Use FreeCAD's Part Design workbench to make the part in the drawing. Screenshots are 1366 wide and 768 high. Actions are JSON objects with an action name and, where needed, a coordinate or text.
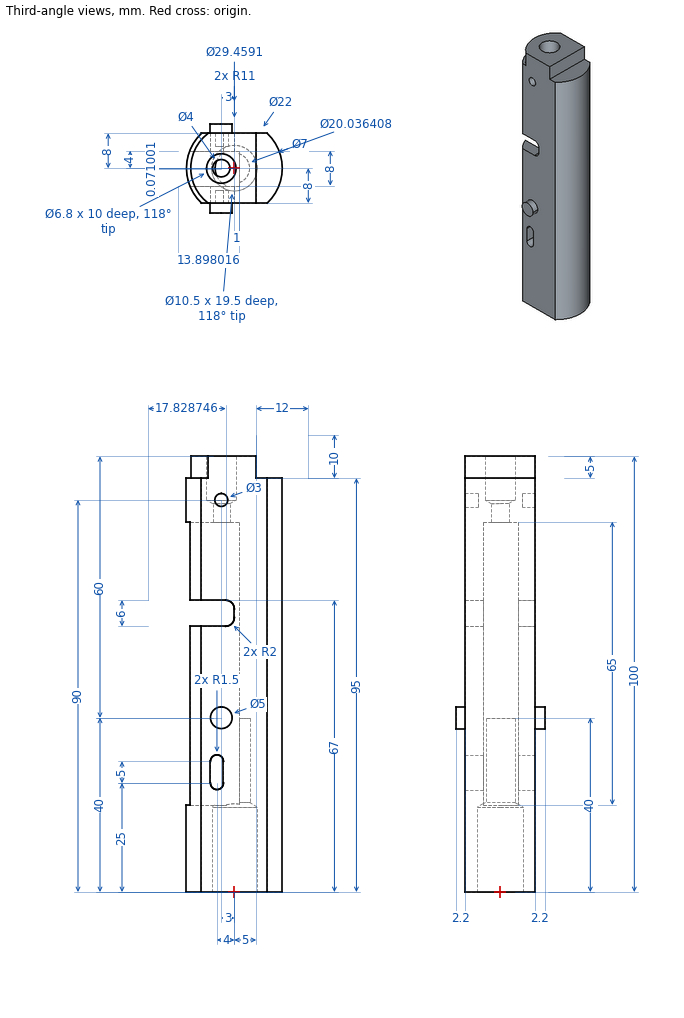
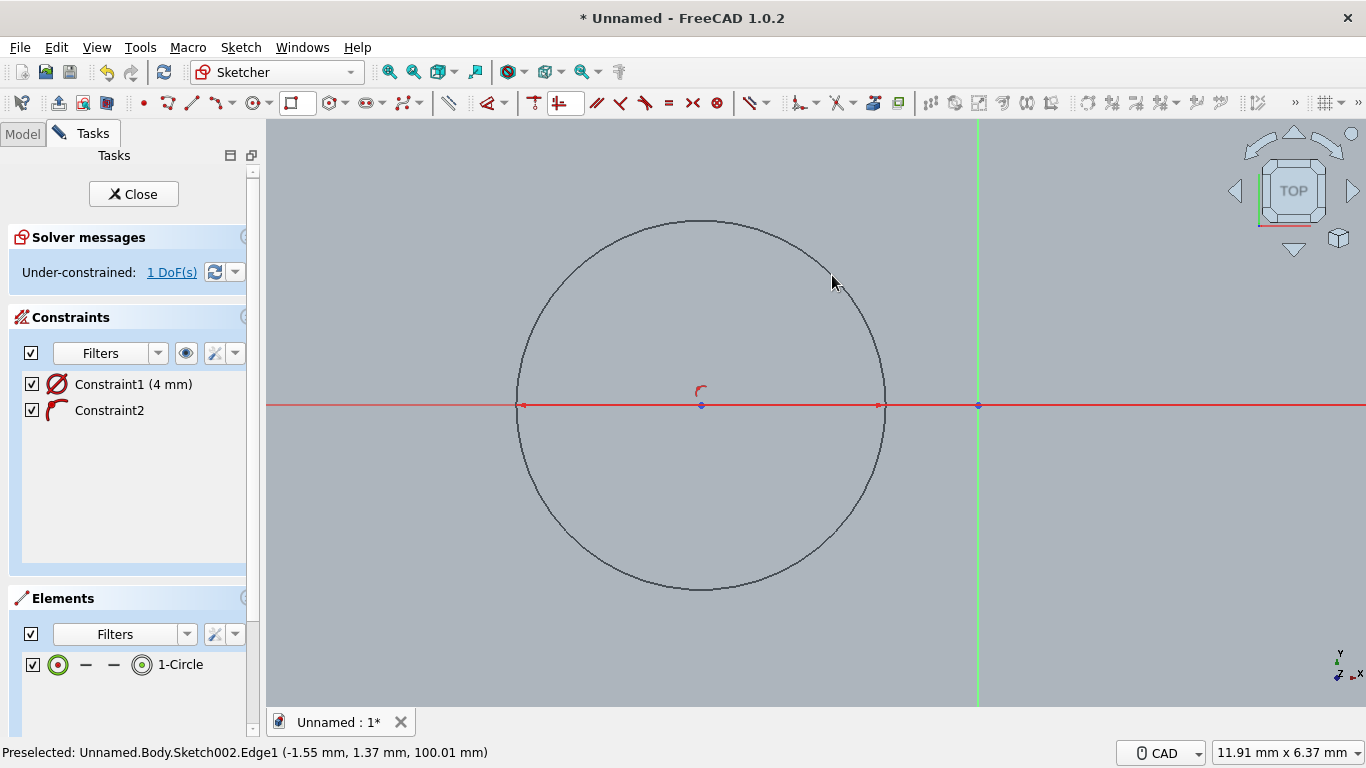
{"action": "key", "text": "d"}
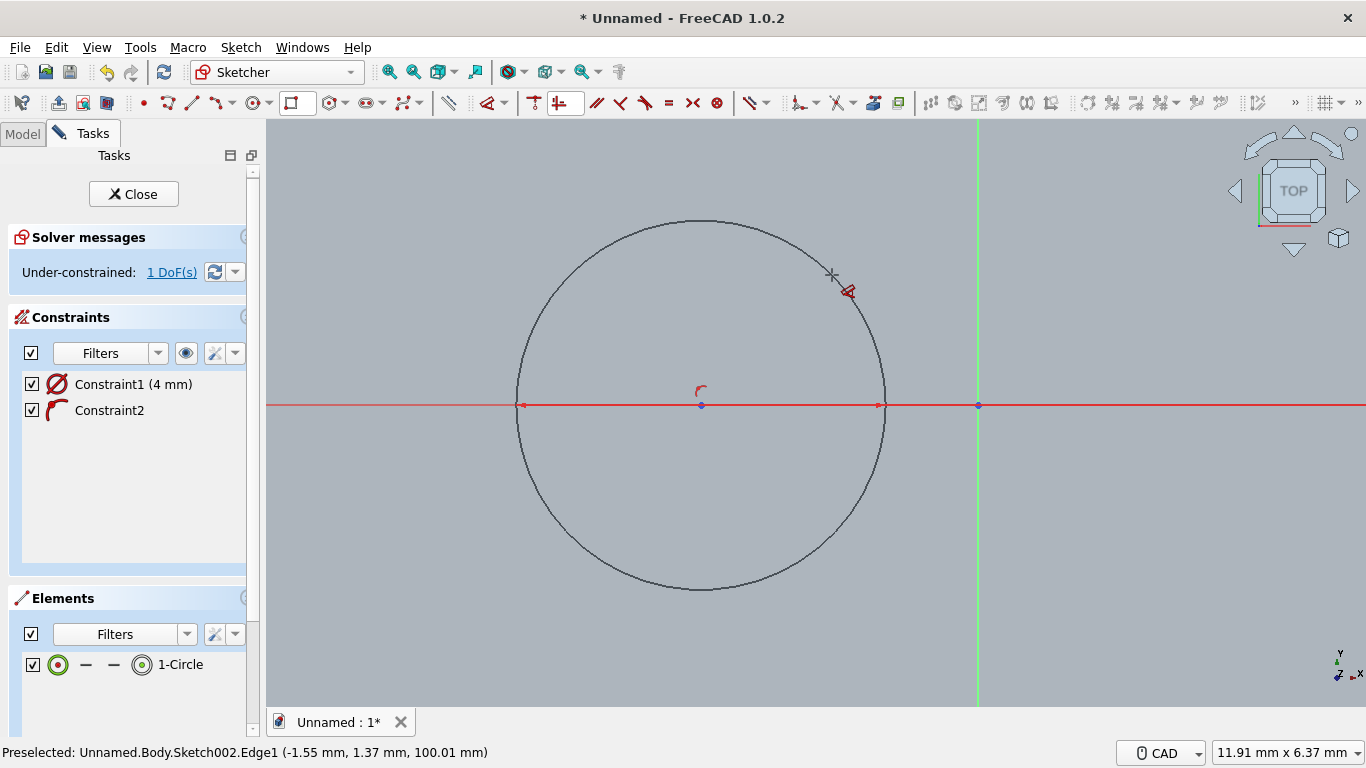
{"action": "left_click", "coordinate": [701, 405]}
{"action": "left_click", "coordinate": [840, 439]}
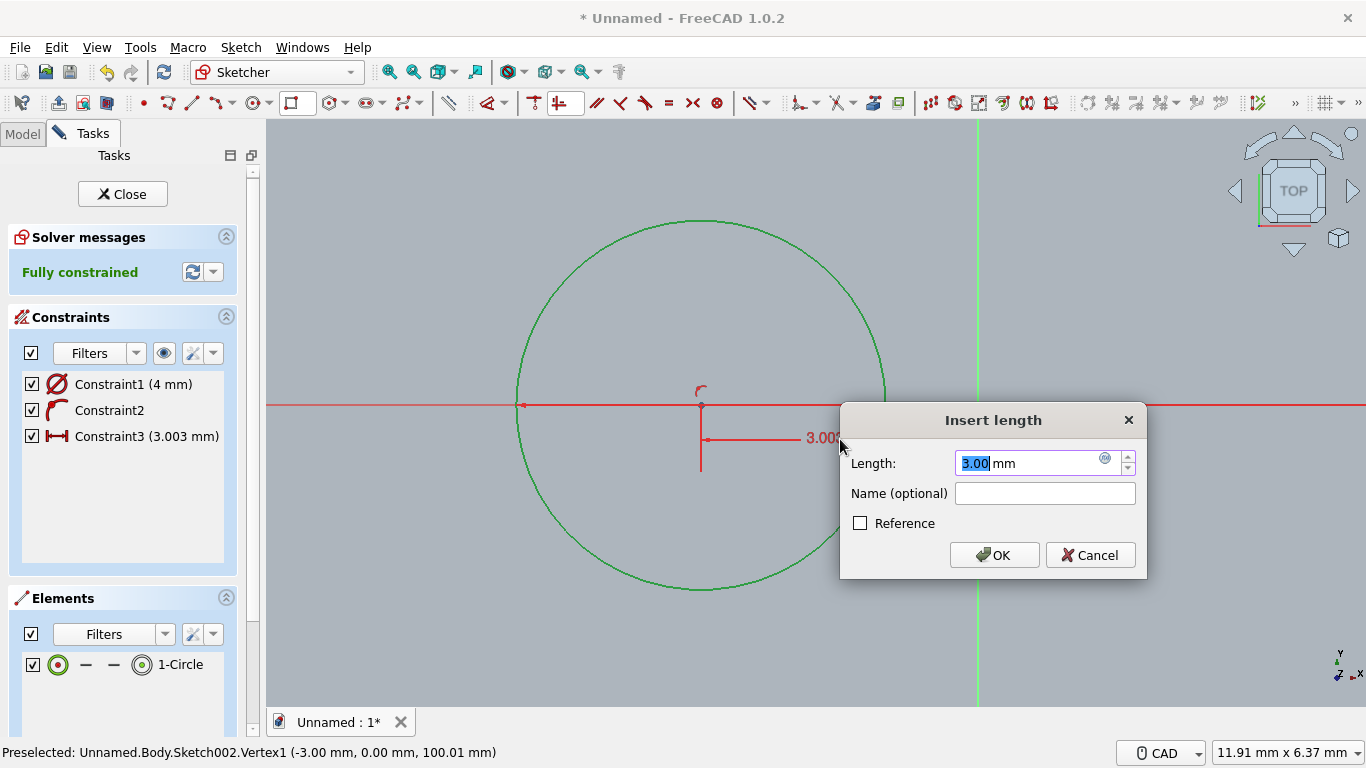
{"action": "type", "text": "3"}
{"action": "key", "text": "Return"}
{"action": "key", "text": "Escape"}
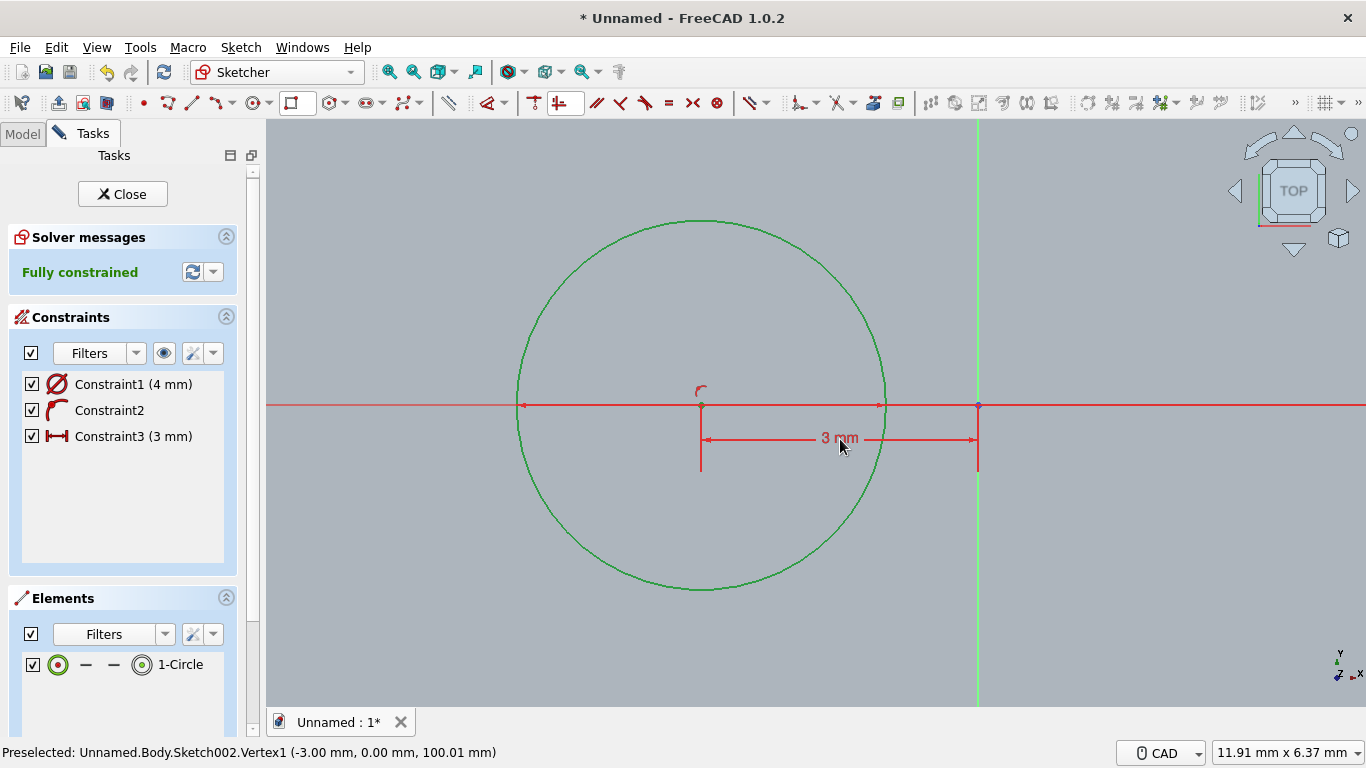
{"action": "left_click", "coordinate": [123, 194]}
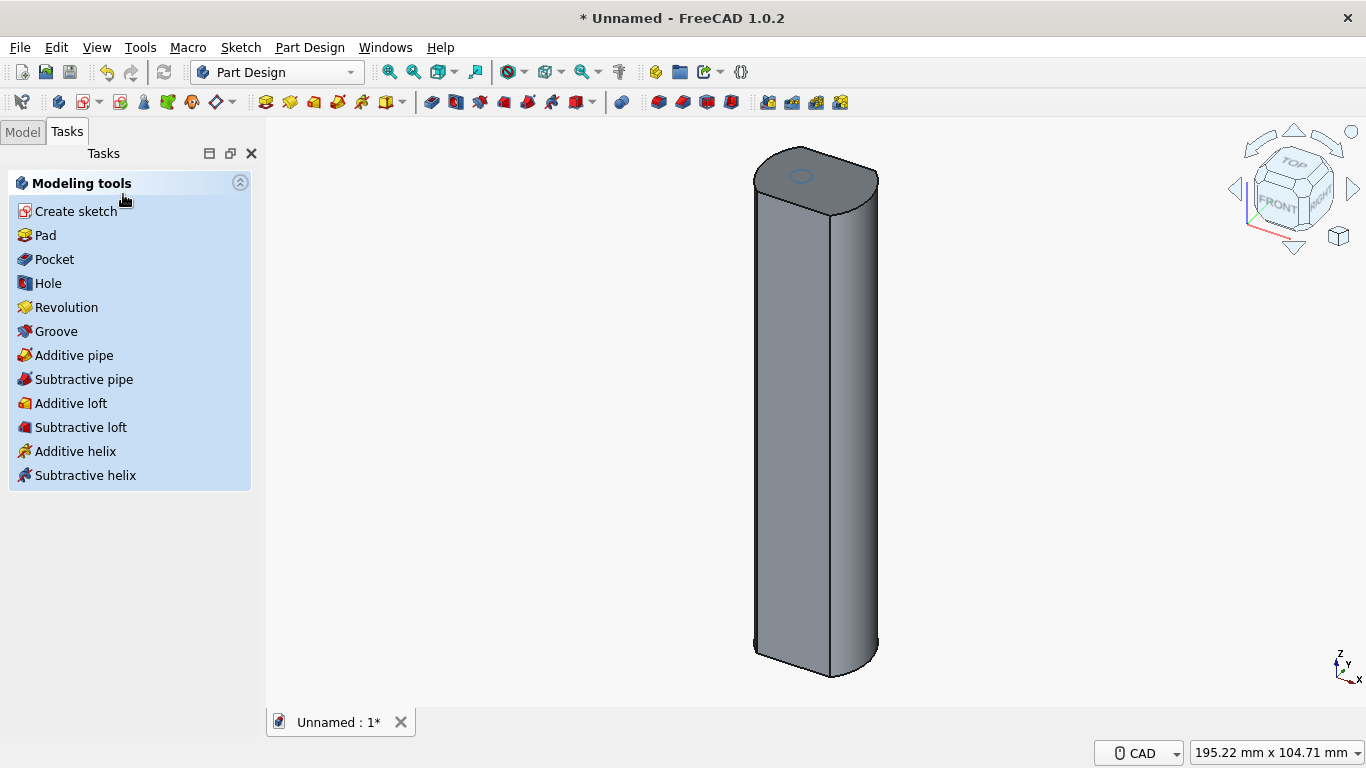
{"action": "left_click", "coordinate": [432, 102]}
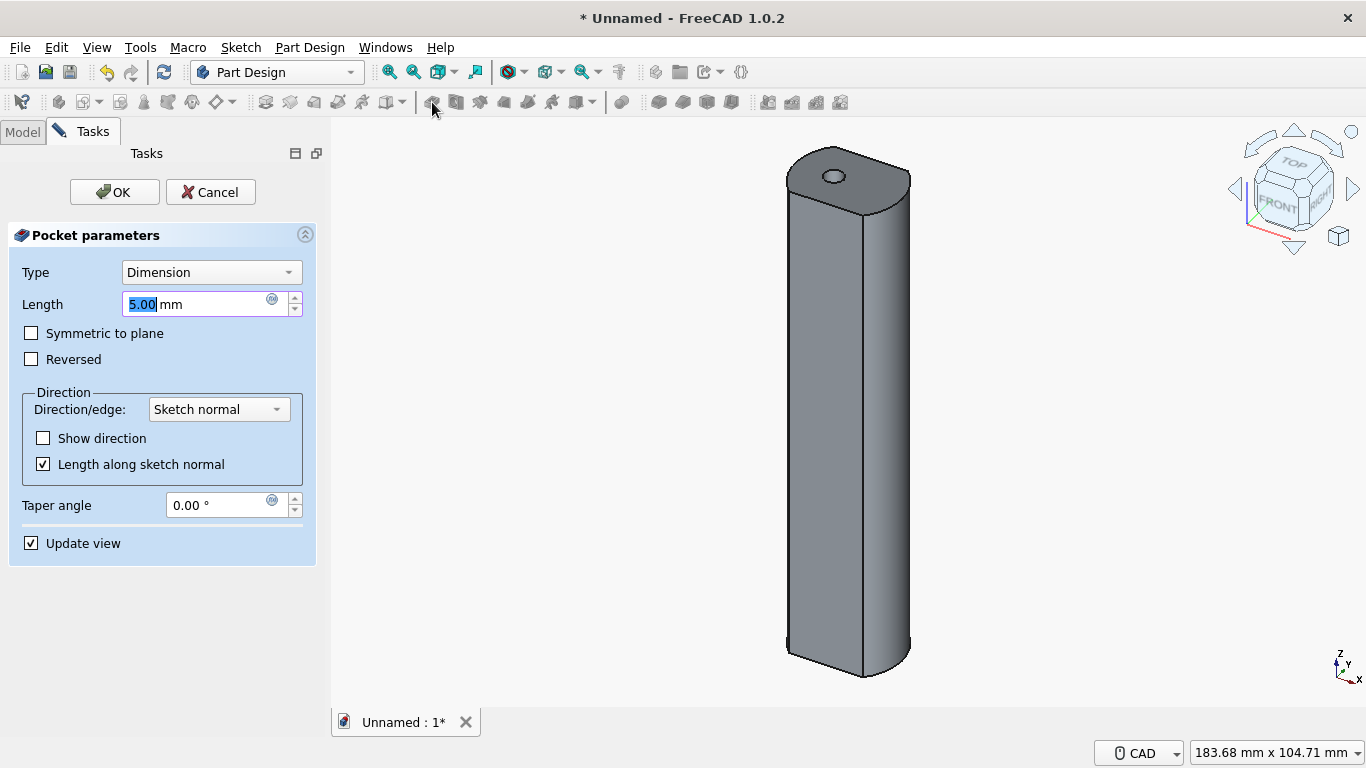
{"action": "type", "text": "60"}
{"action": "key", "text": "Tab"}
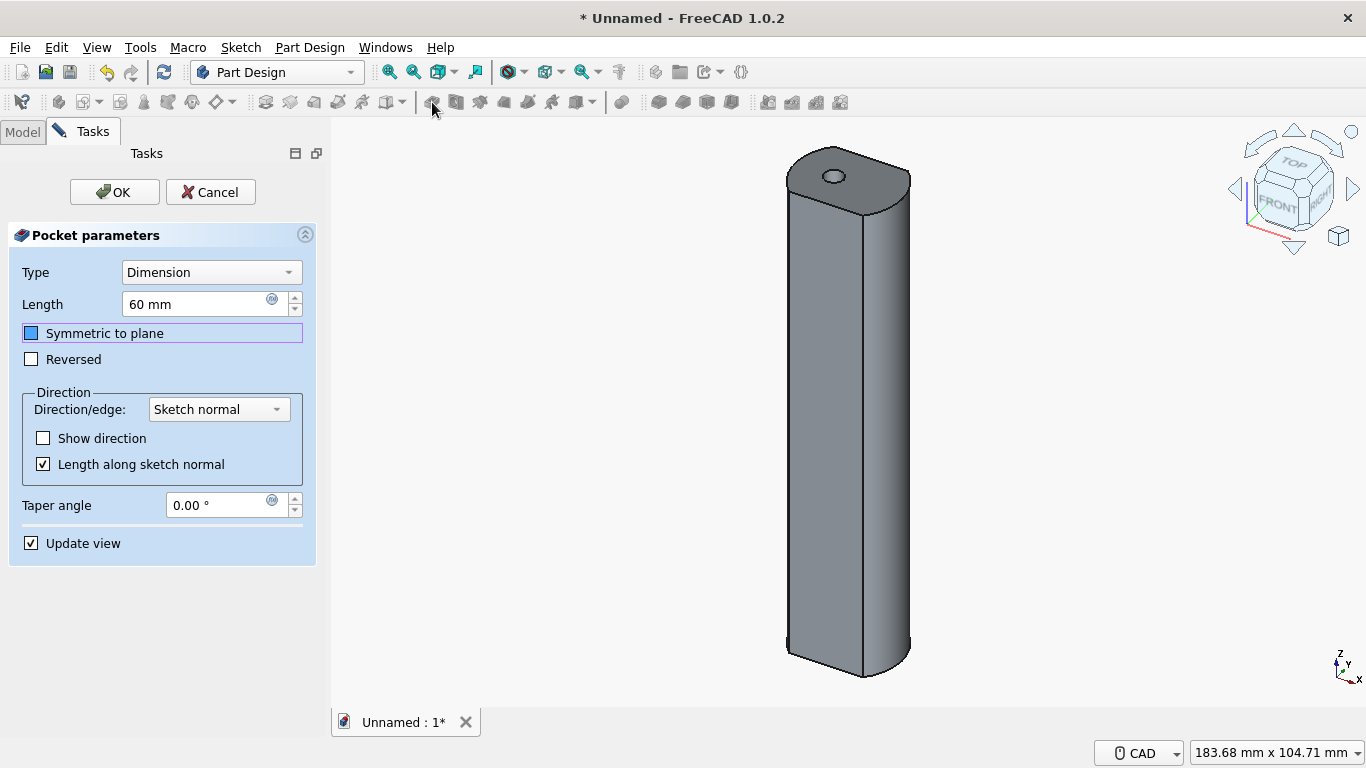
{"action": "left_click", "coordinate": [115, 192]}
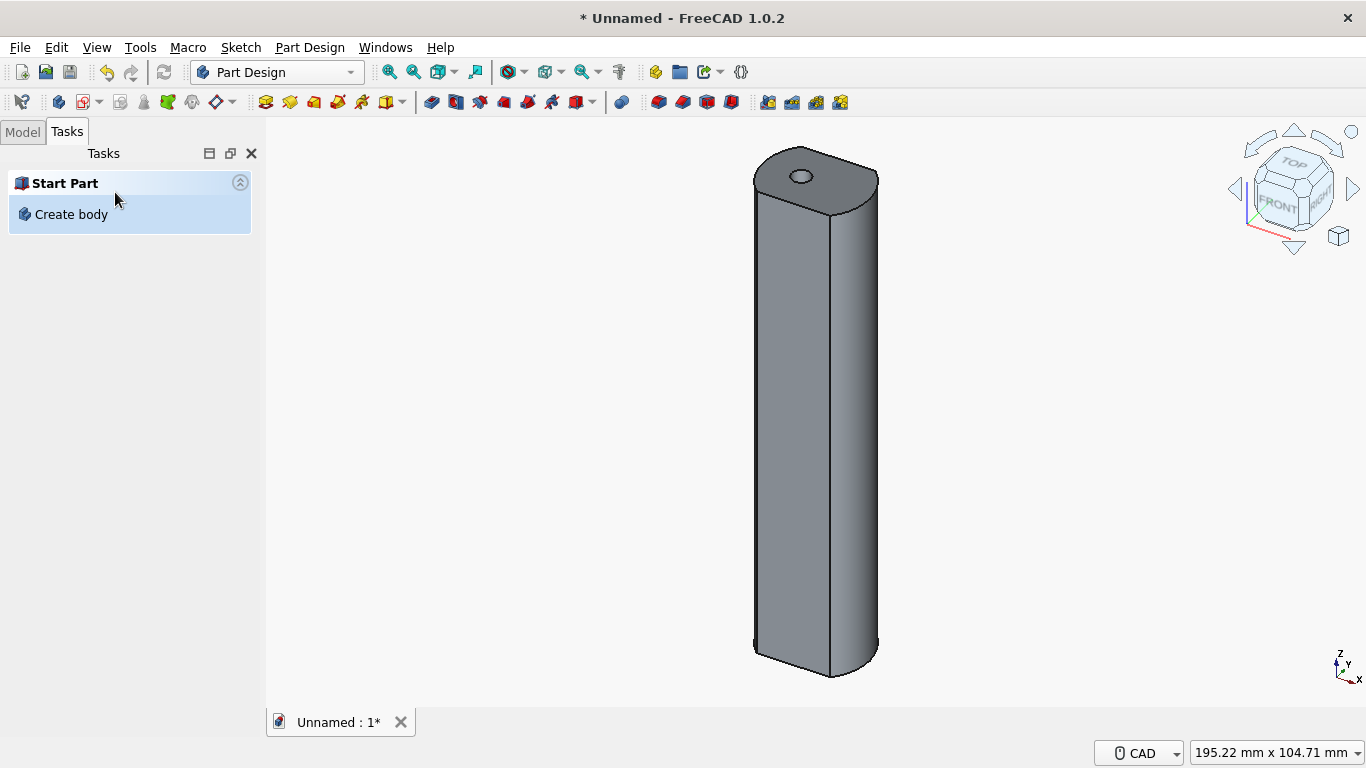
{"action": "left_click", "coordinate": [23, 131]}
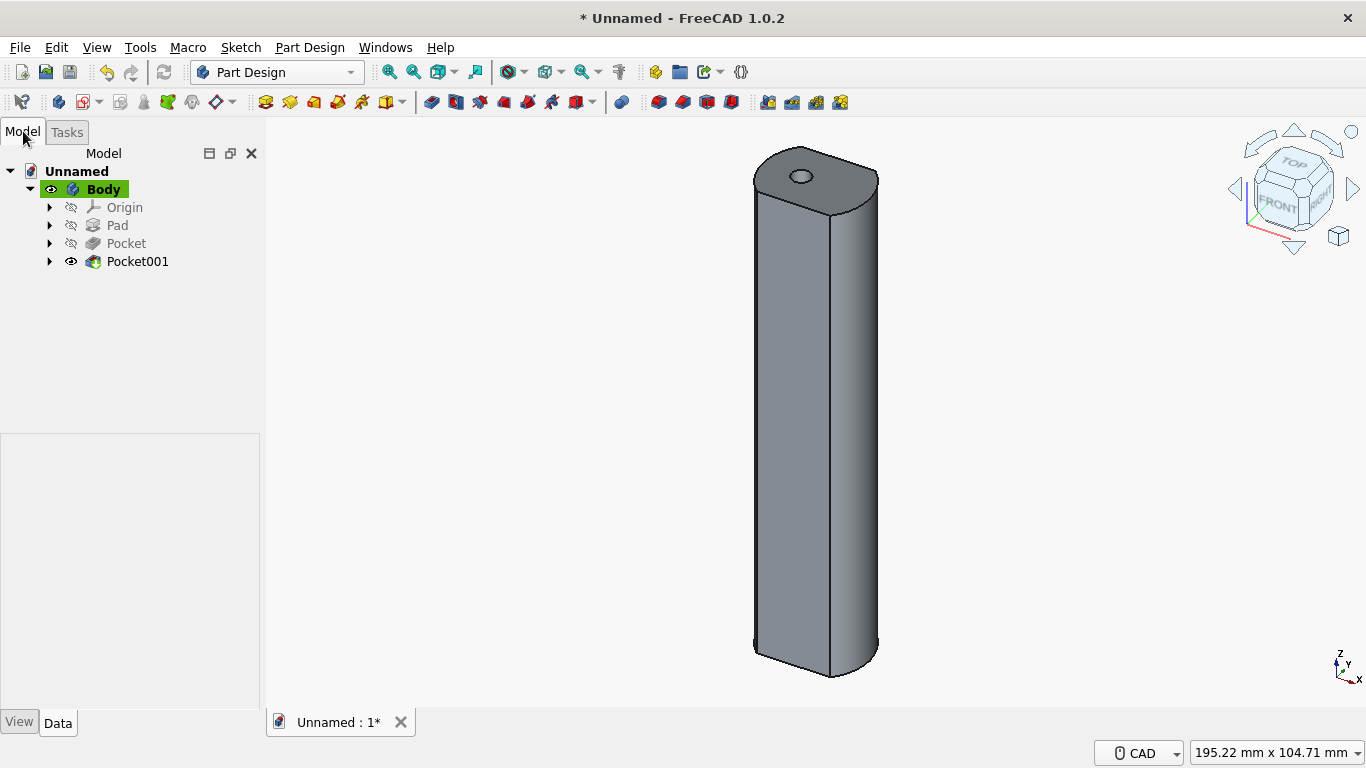
{"action": "left_click", "coordinate": [50, 207]}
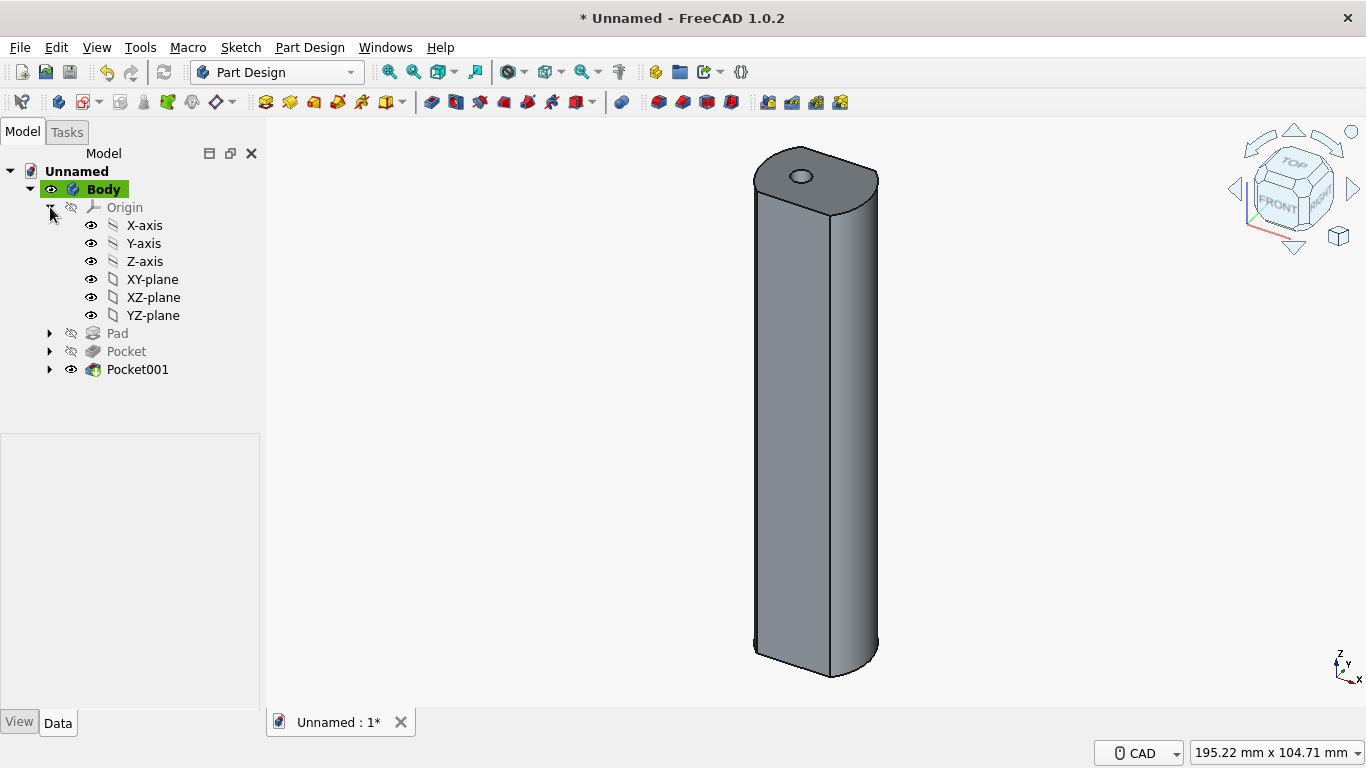
{"action": "left_click", "coordinate": [136, 279]}